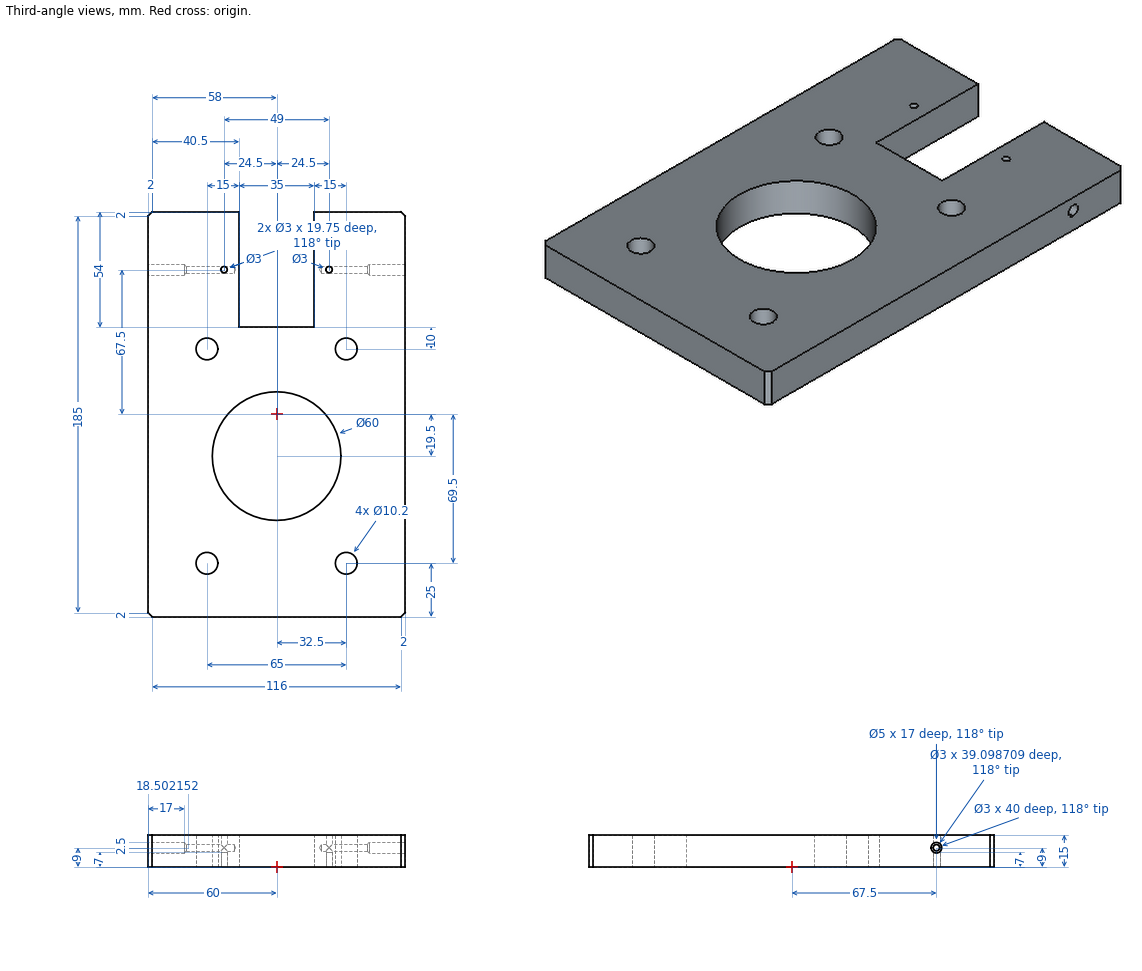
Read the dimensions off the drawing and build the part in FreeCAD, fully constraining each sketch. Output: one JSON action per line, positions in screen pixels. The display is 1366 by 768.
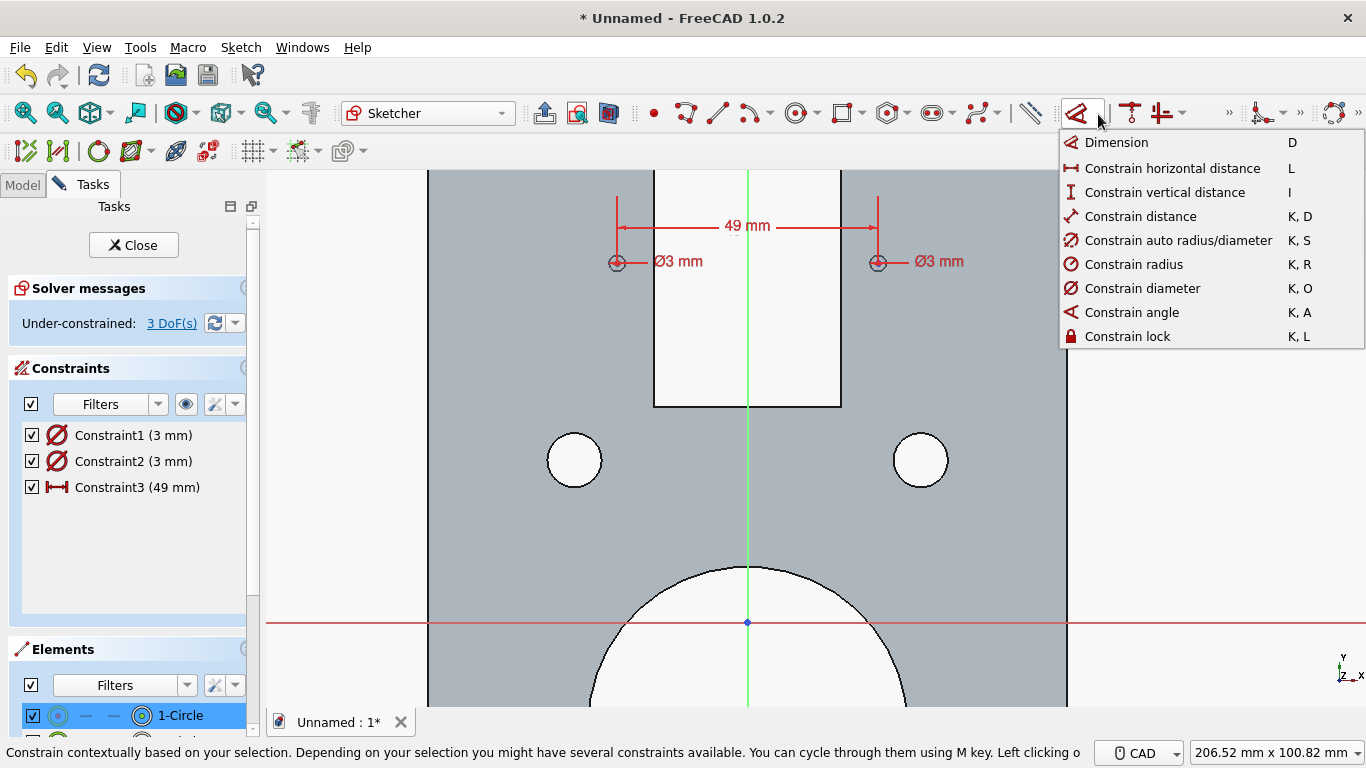
{"action": "left_click", "coordinate": [1212, 168]}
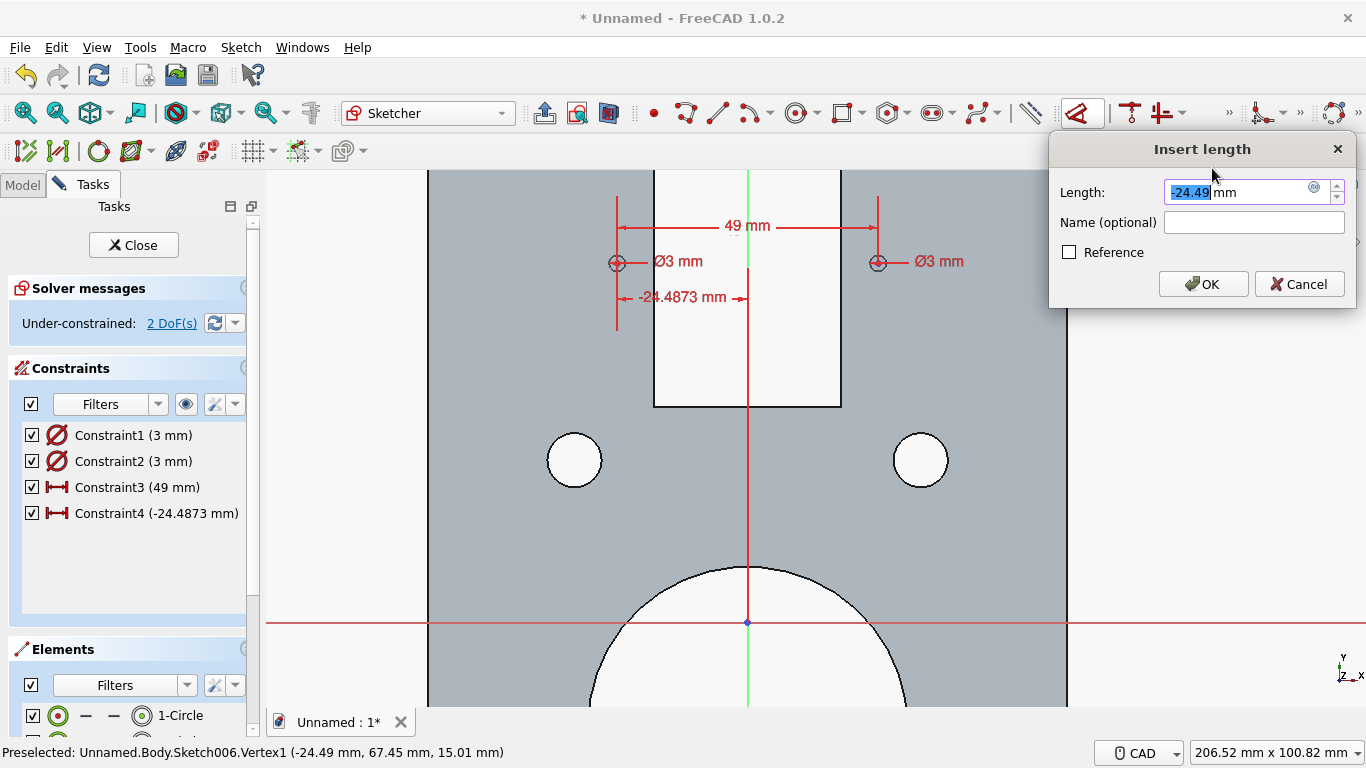
{"action": "type", "text": "-24.5"}
{"action": "key", "text": "Return"}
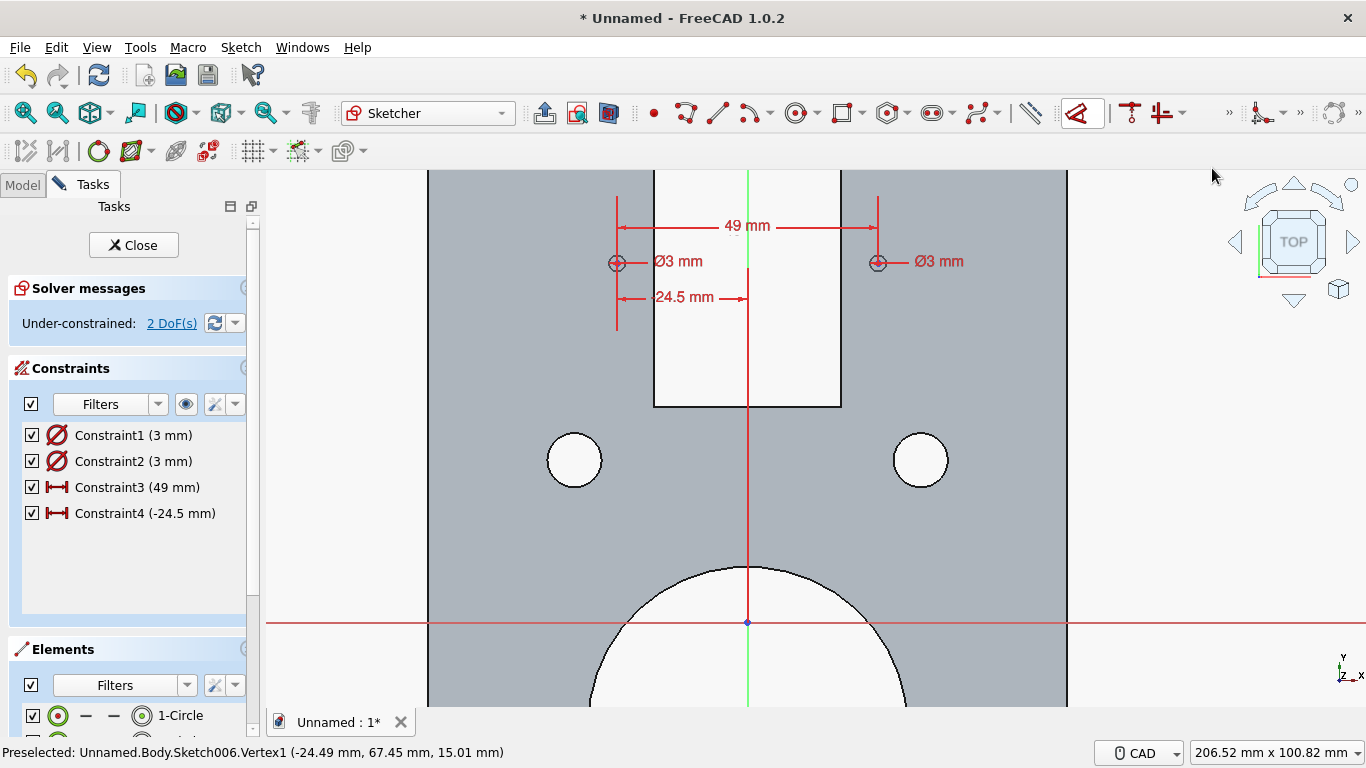
{"action": "left_click", "coordinate": [617, 263]}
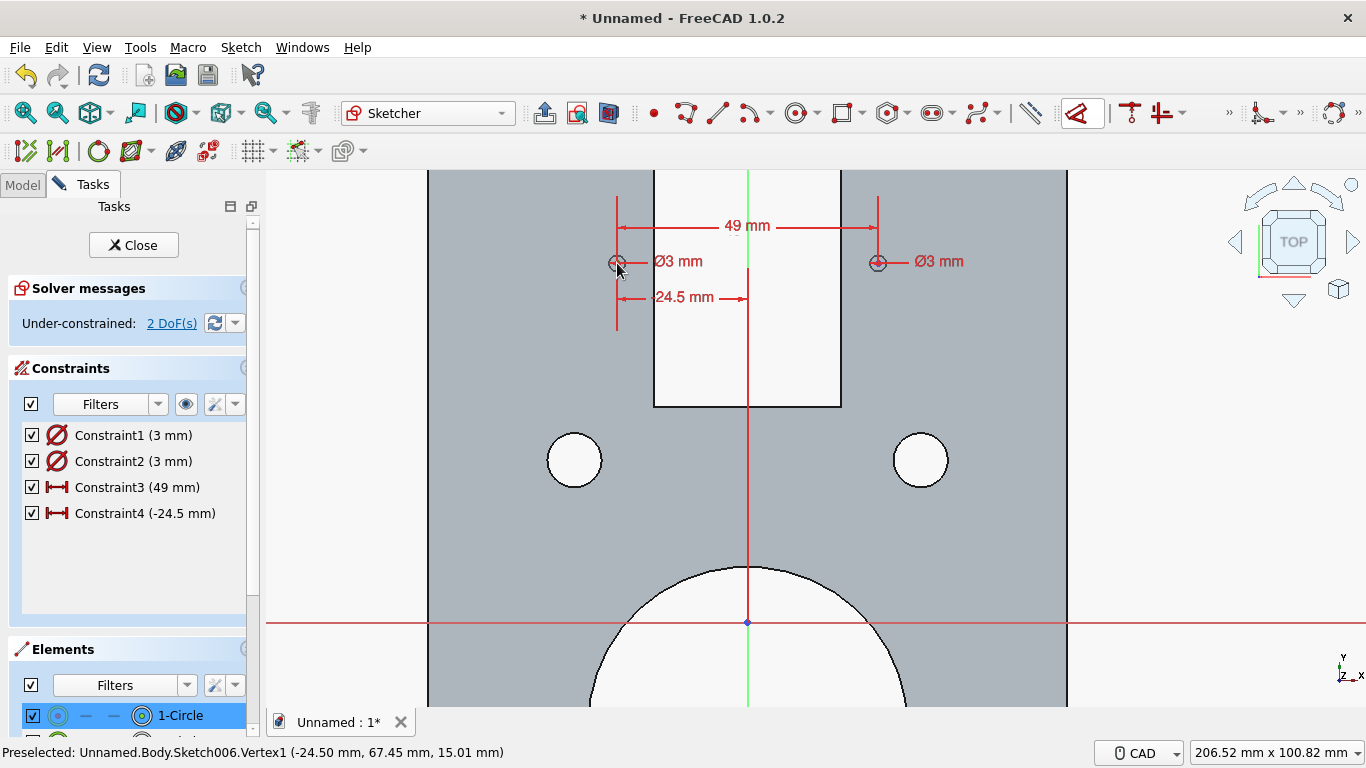
{"action": "left_click", "coordinate": [1098, 114]}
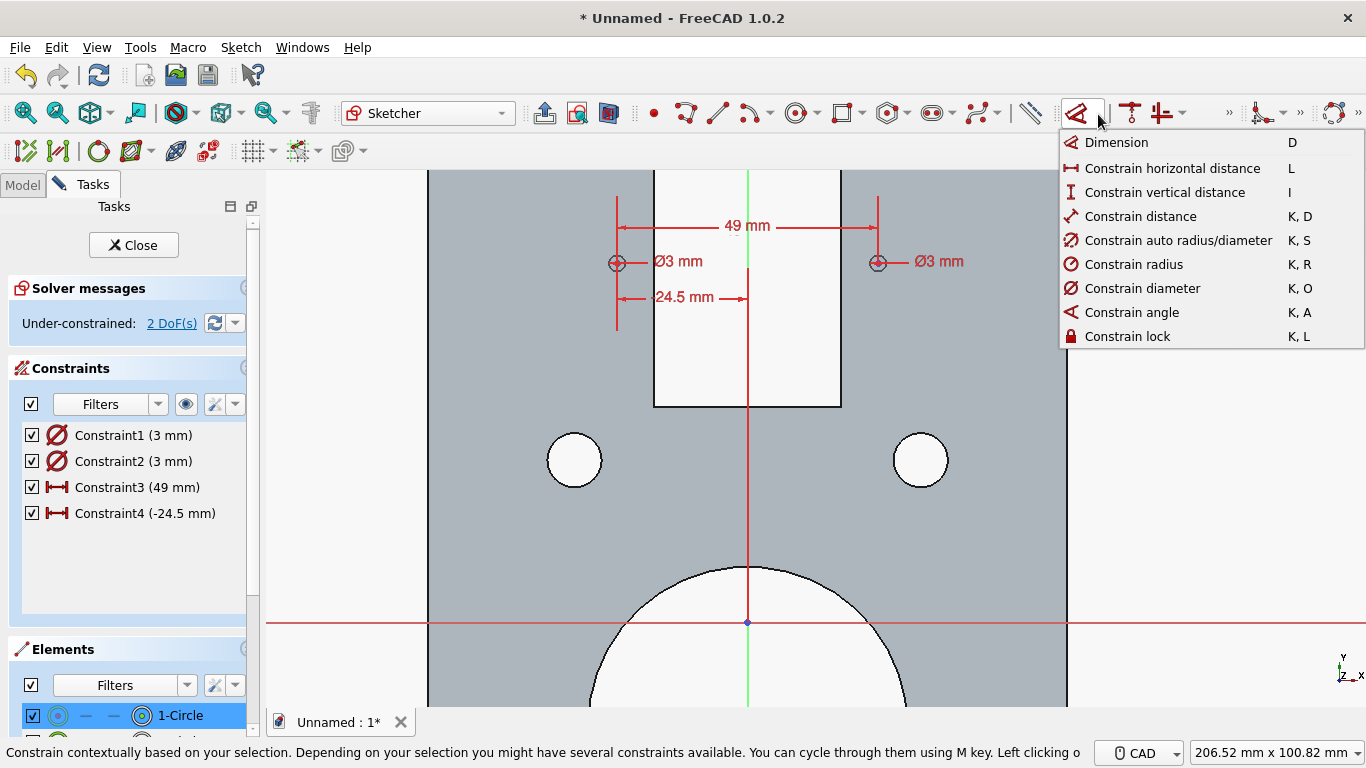
{"action": "left_click", "coordinate": [1212, 192]}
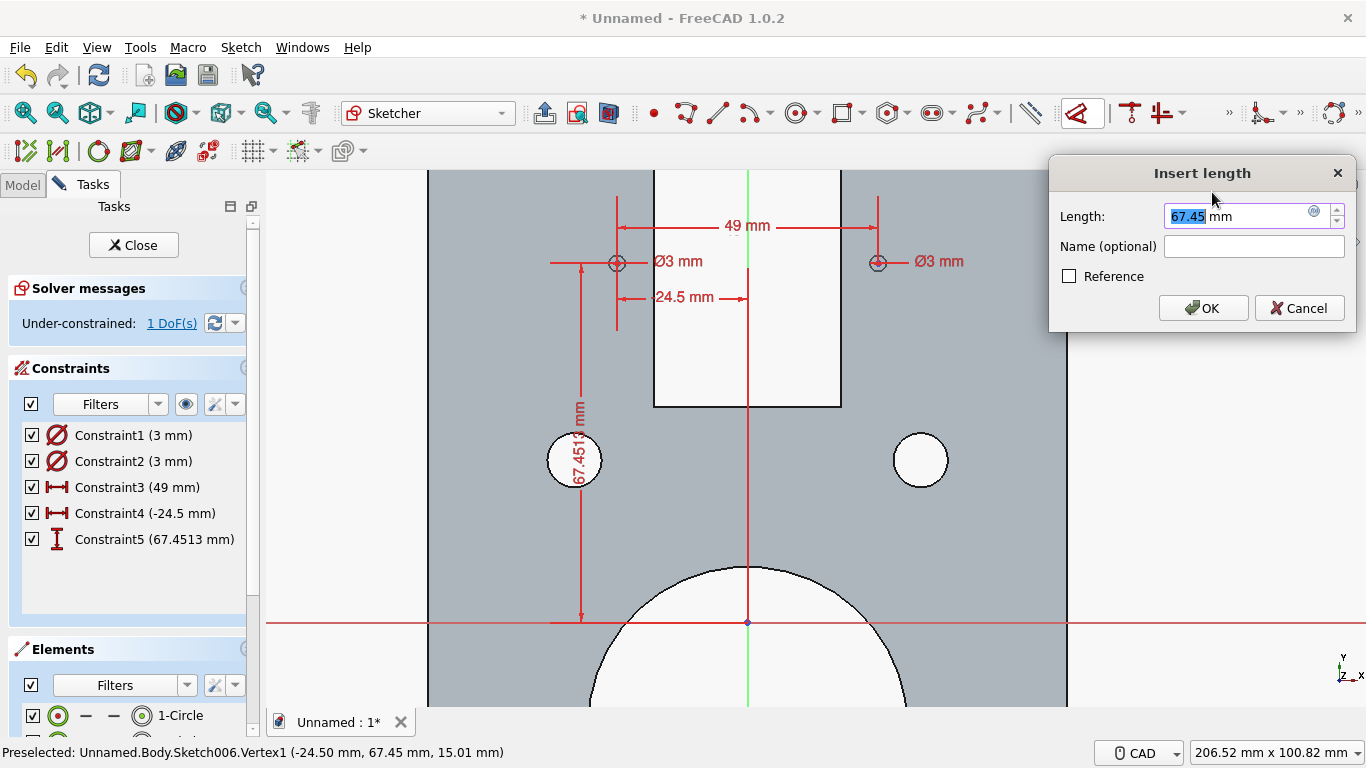
{"action": "type", "text": "67.5"}
{"action": "key", "text": "Return"}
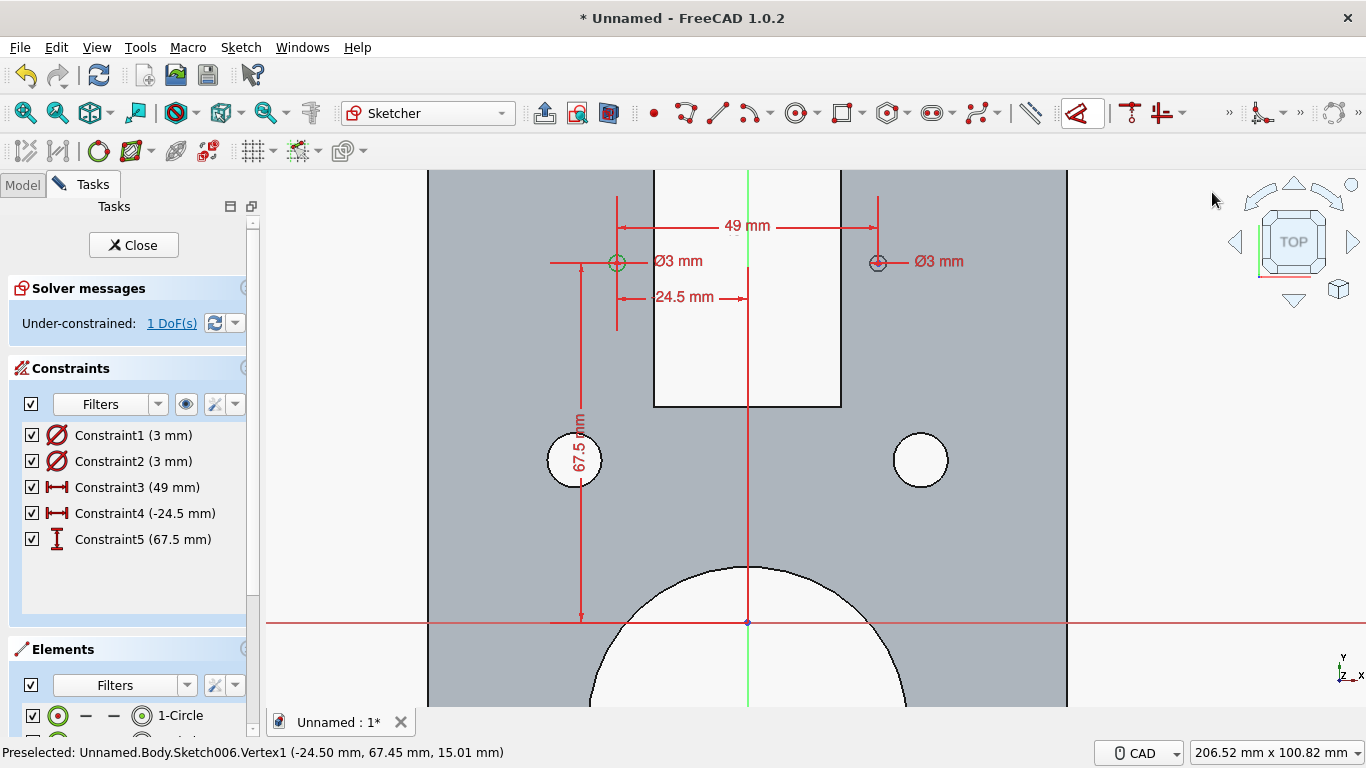
{"action": "left_click", "coordinate": [878, 263]}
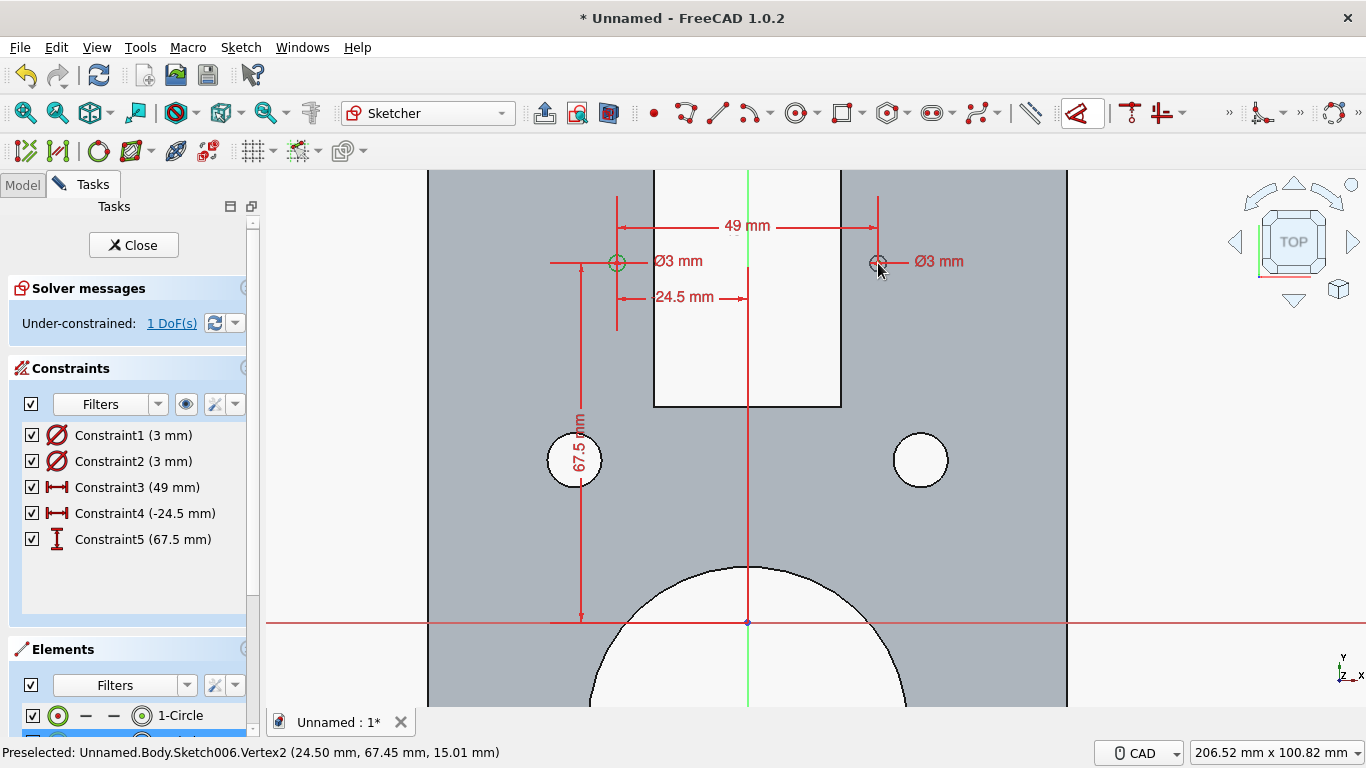
{"action": "key", "text": "i"}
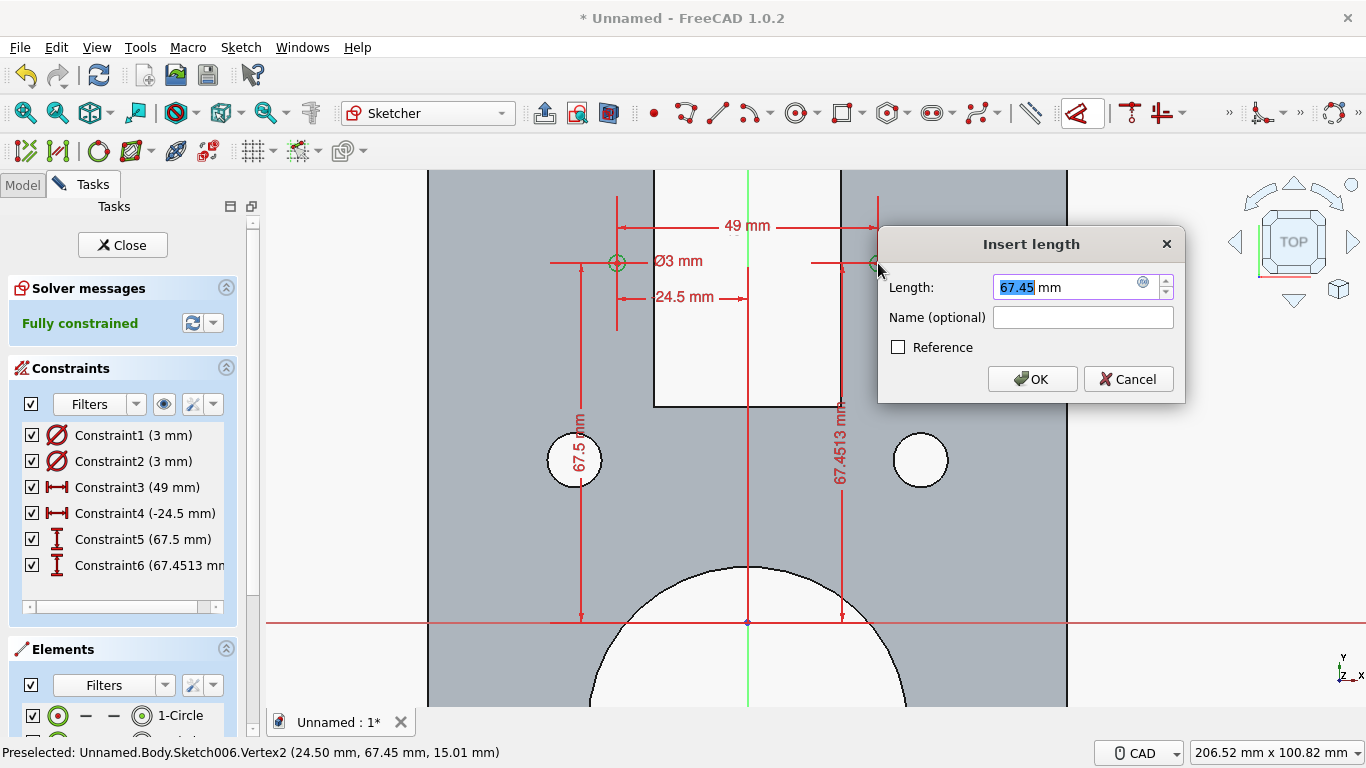
{"action": "type", "text": "67.5"}
{"action": "key", "text": "Return"}